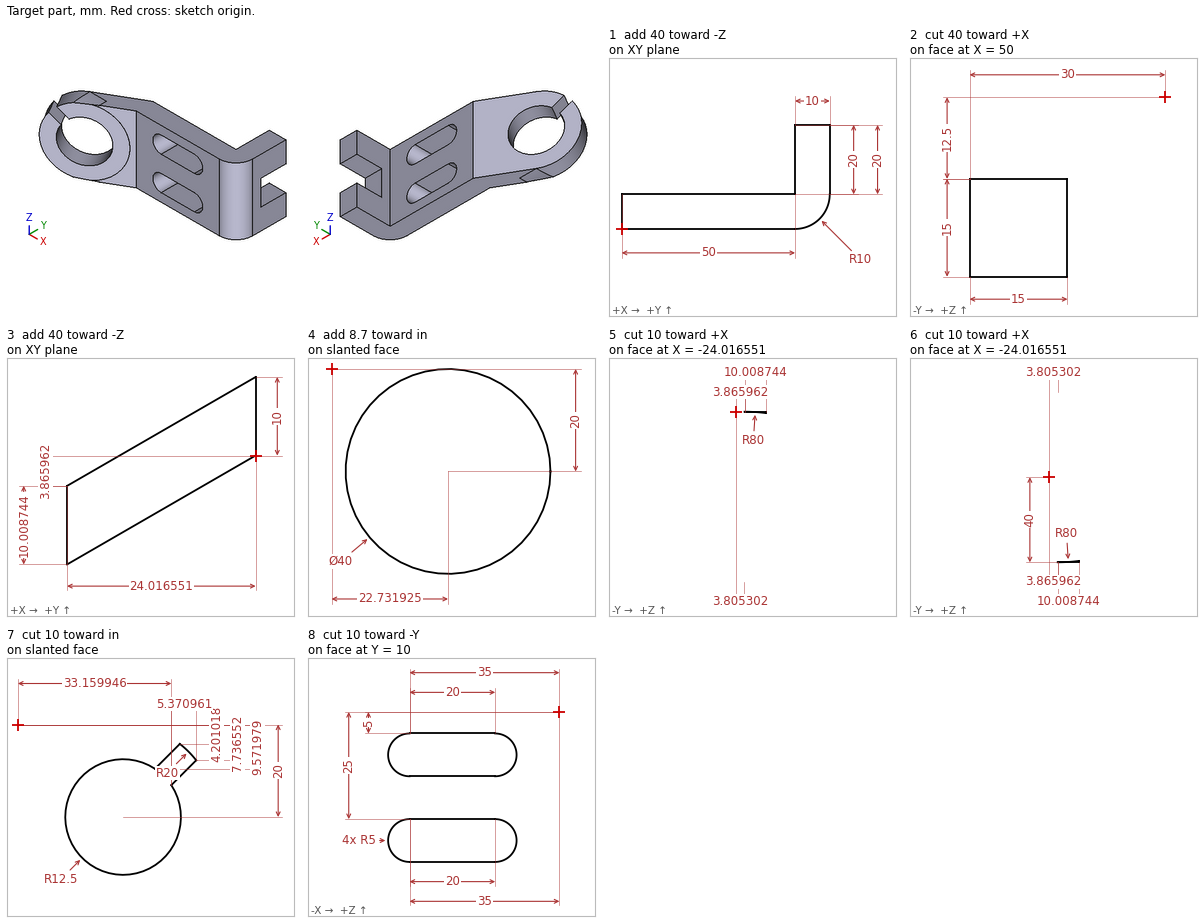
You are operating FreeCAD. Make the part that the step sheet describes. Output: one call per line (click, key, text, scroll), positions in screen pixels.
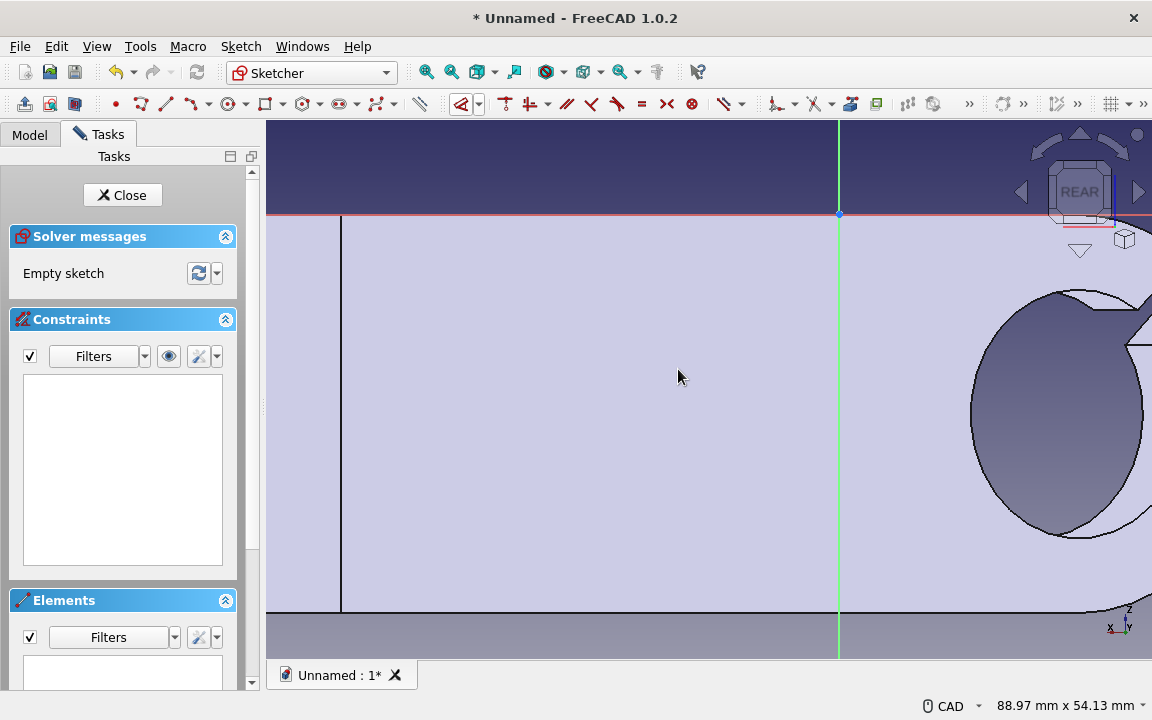
click(338, 104)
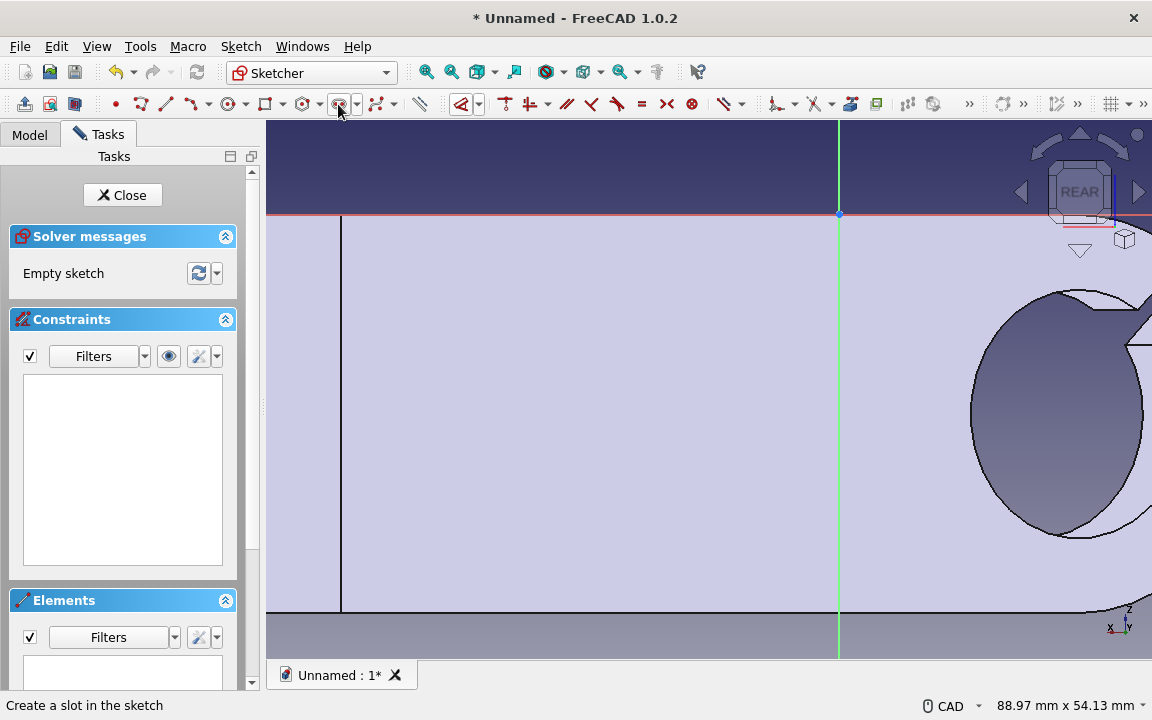
click(491, 514)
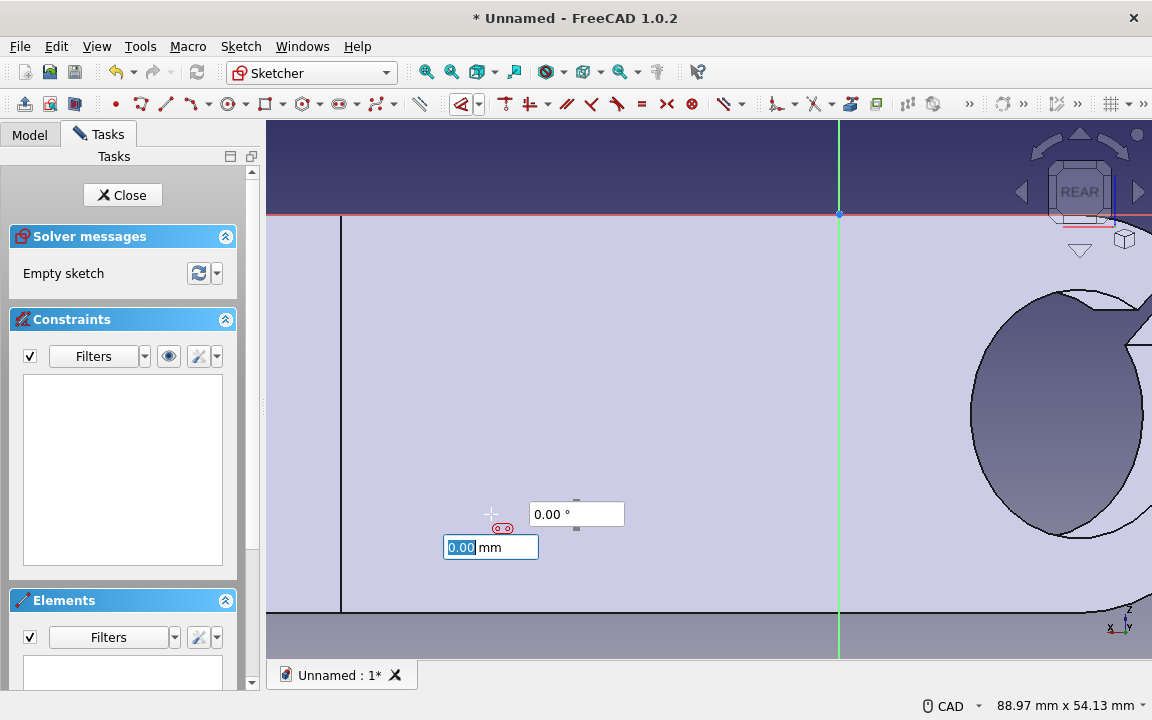
click(690, 514)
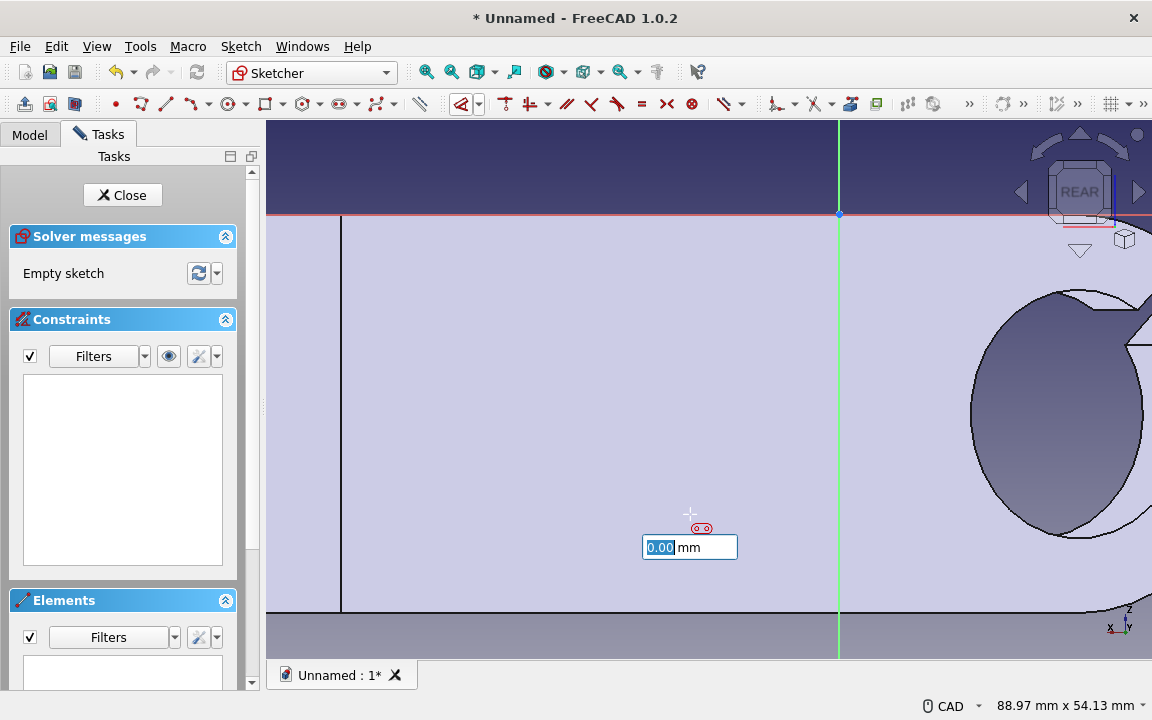
click(590, 464)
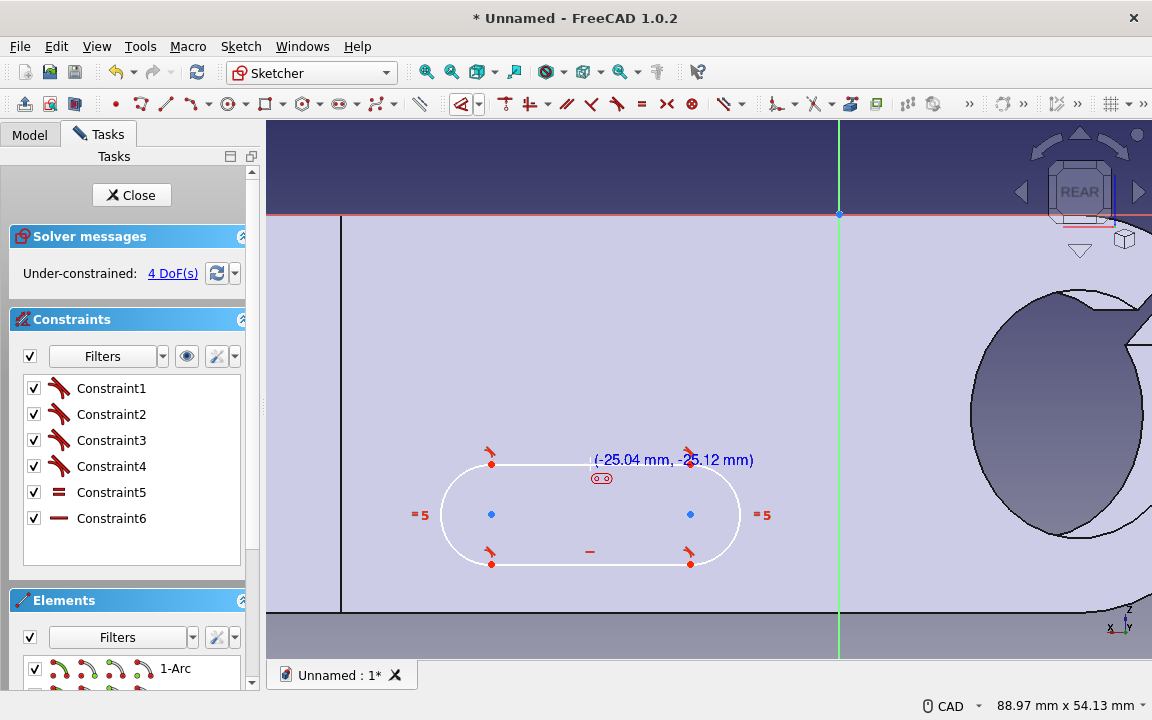
click(491, 314)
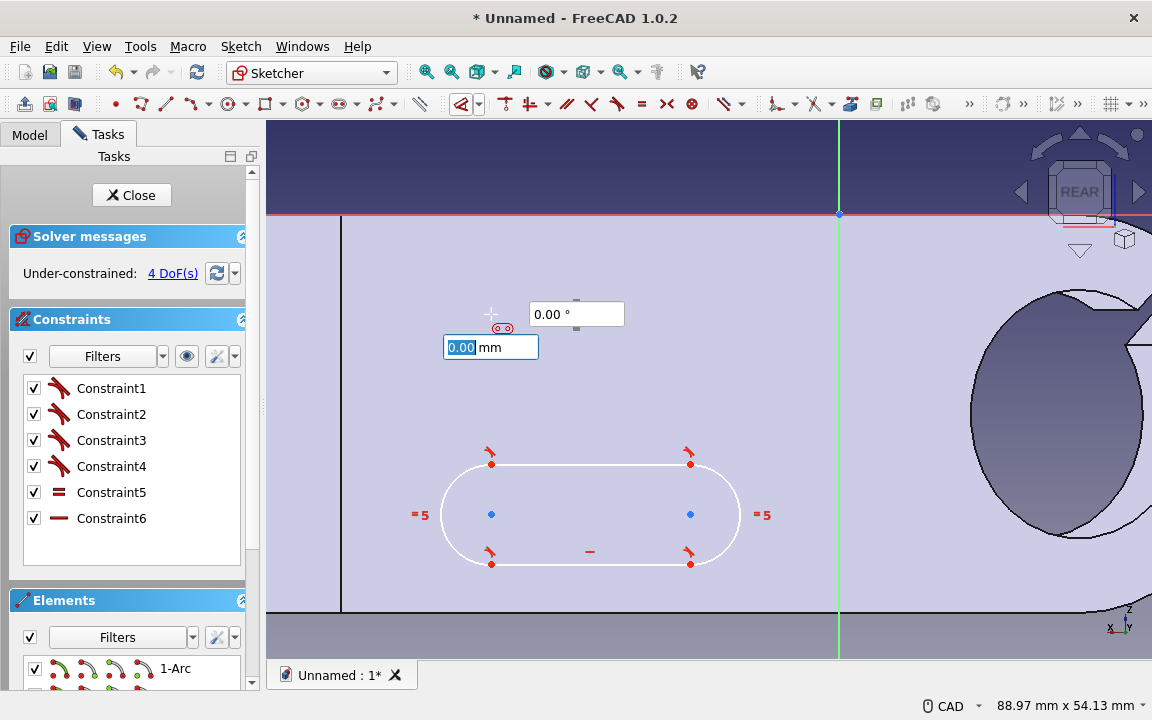
click(690, 314)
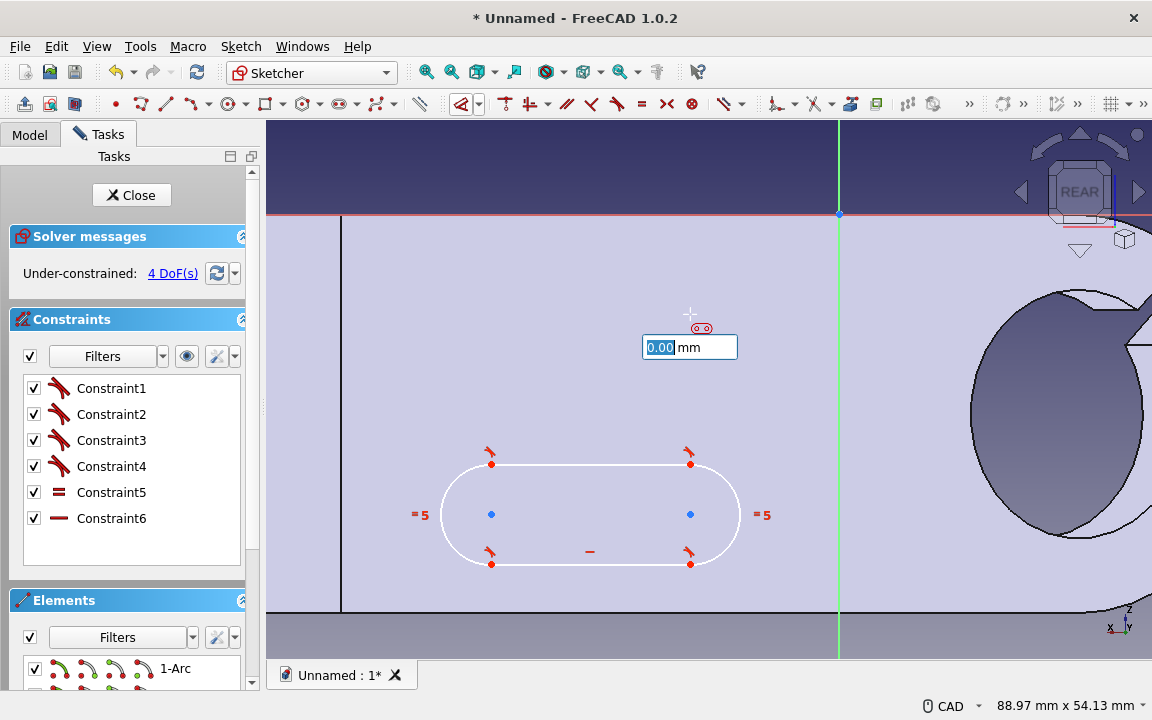
click(590, 265)
key(Escape)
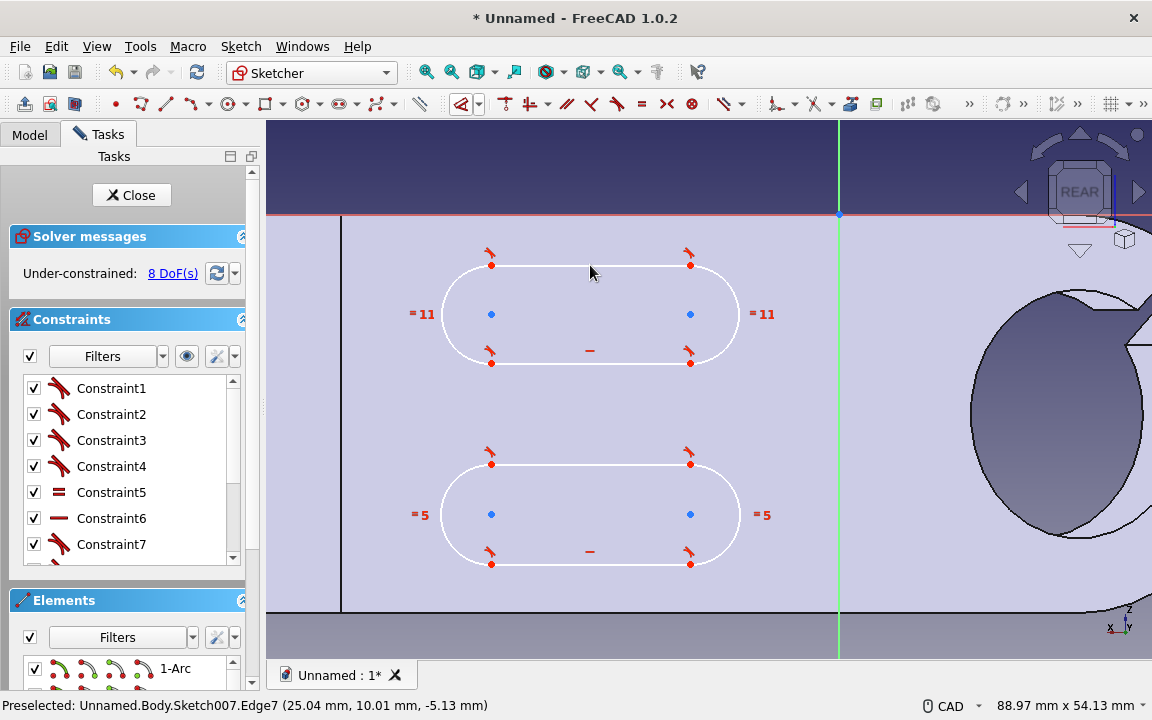
click(451, 486)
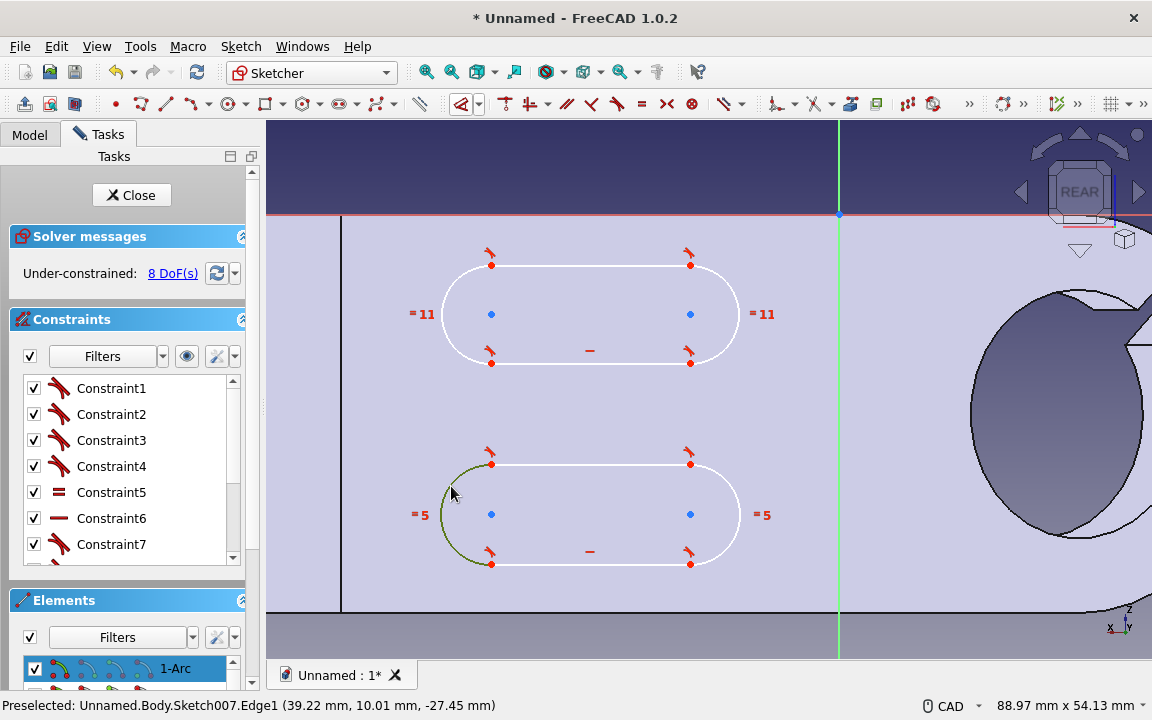
click(451, 286)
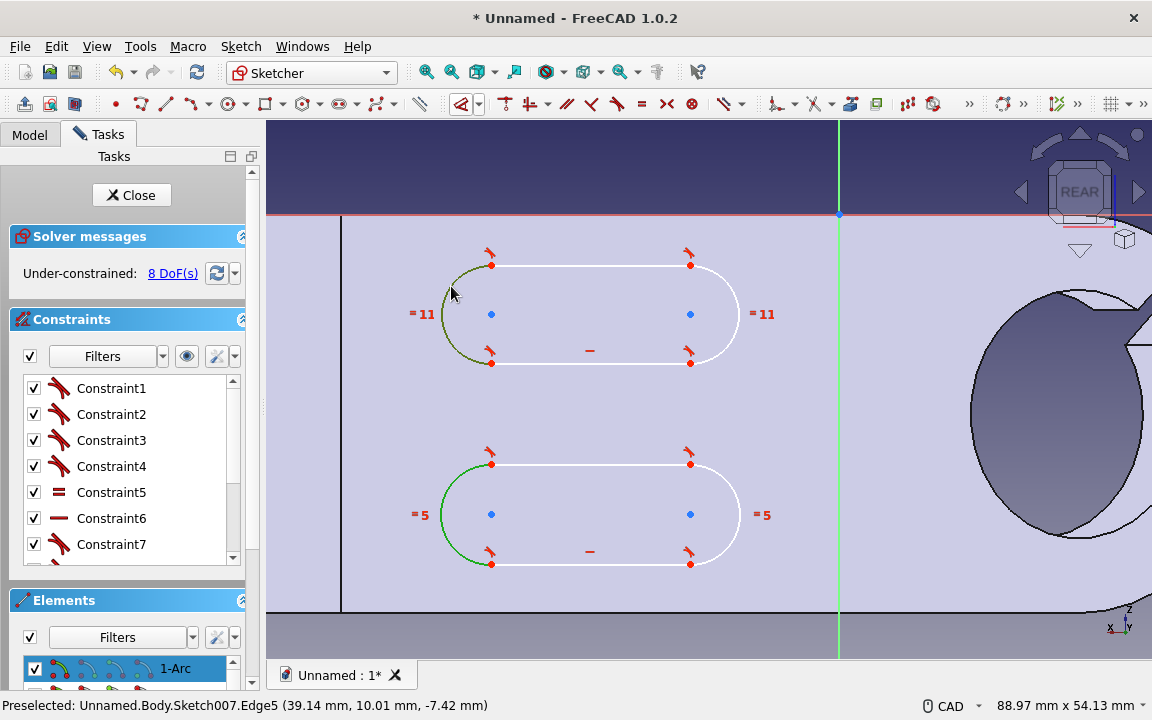
click(642, 104)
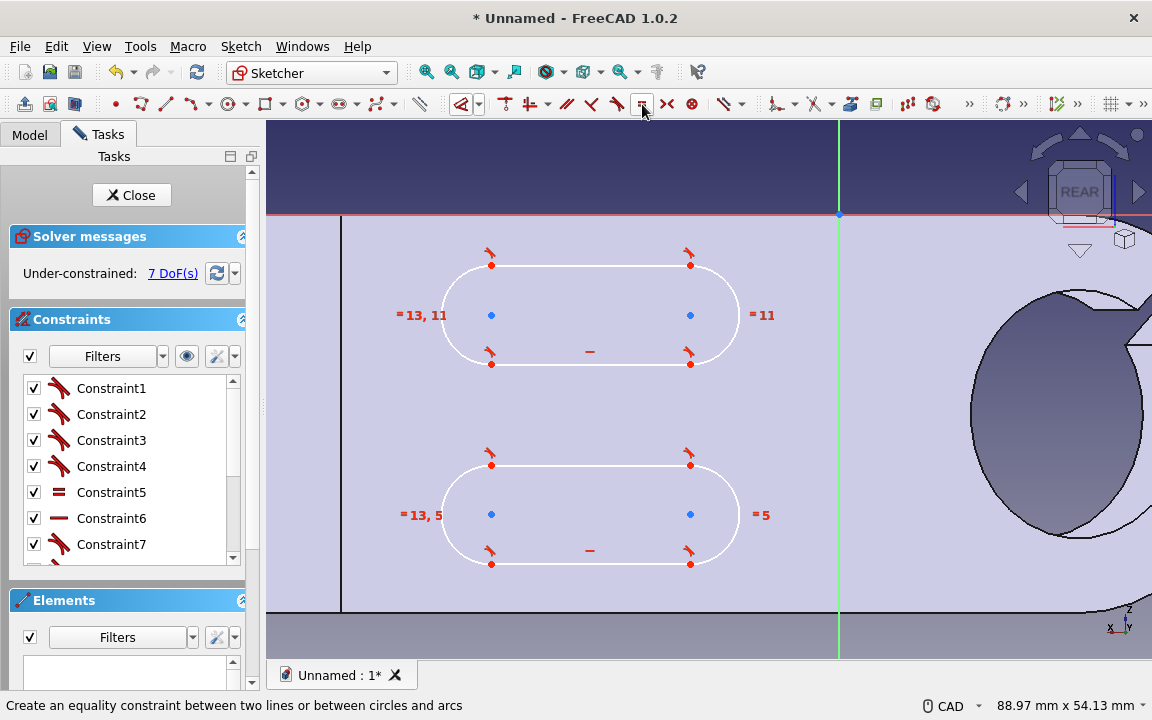
click(451, 486)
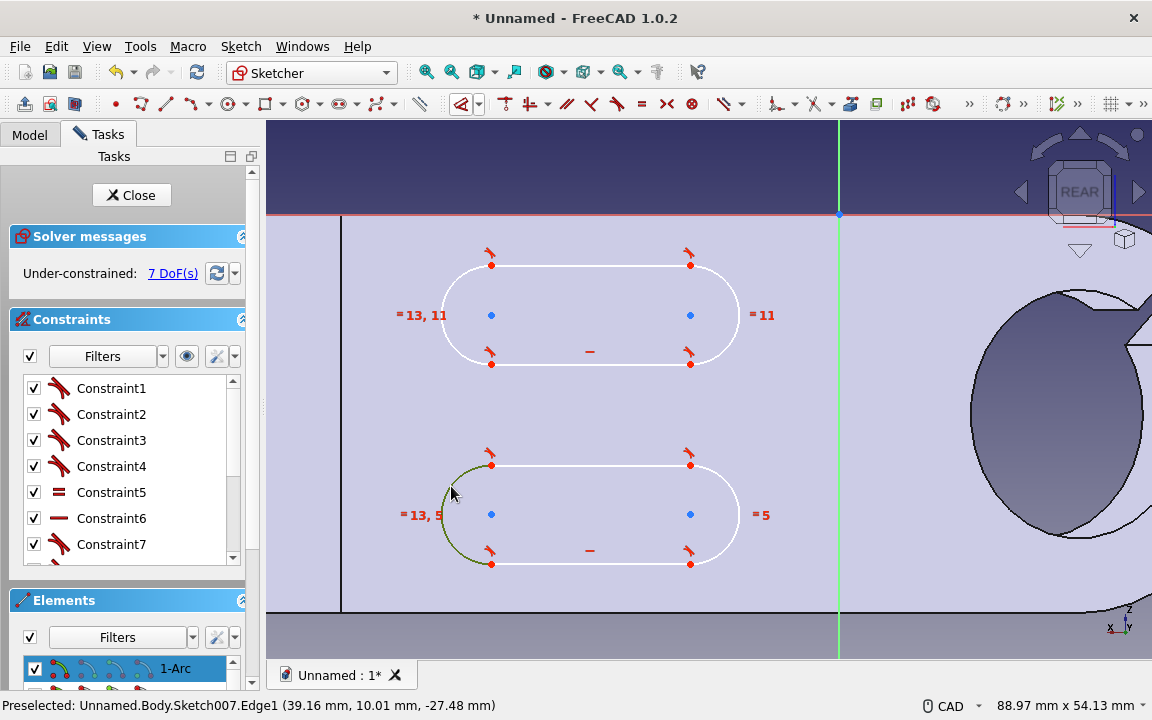
key(k)
key(r)